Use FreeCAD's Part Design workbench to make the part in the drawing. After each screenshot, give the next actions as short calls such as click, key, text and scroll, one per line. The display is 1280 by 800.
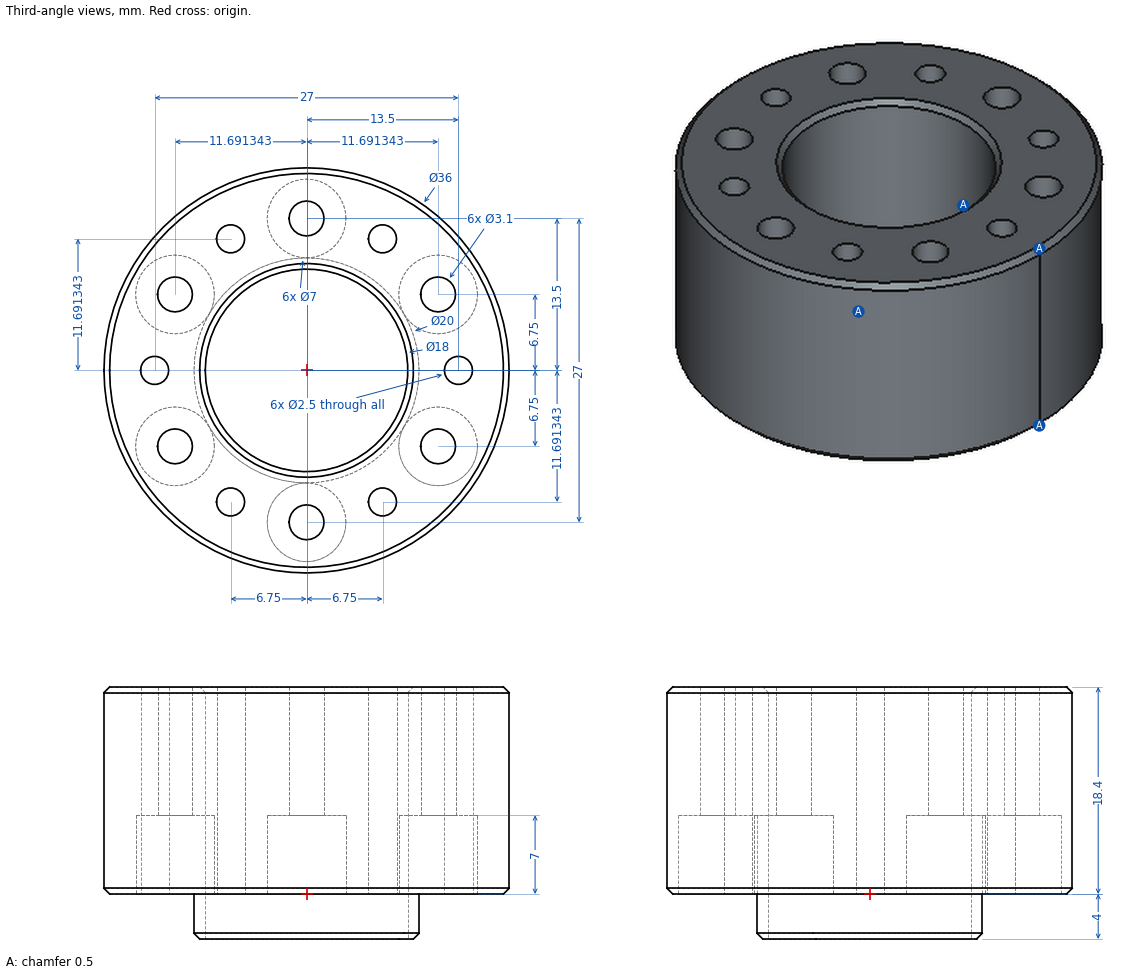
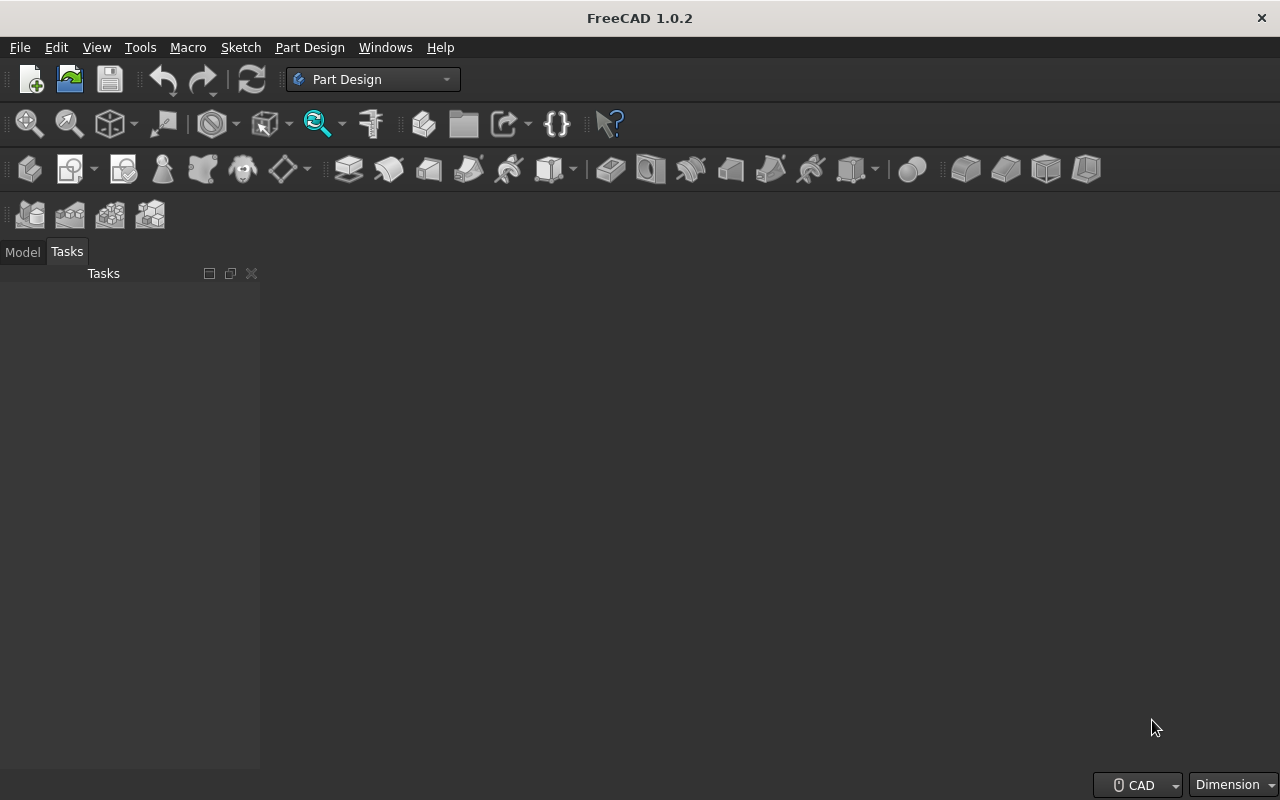
click(30, 80)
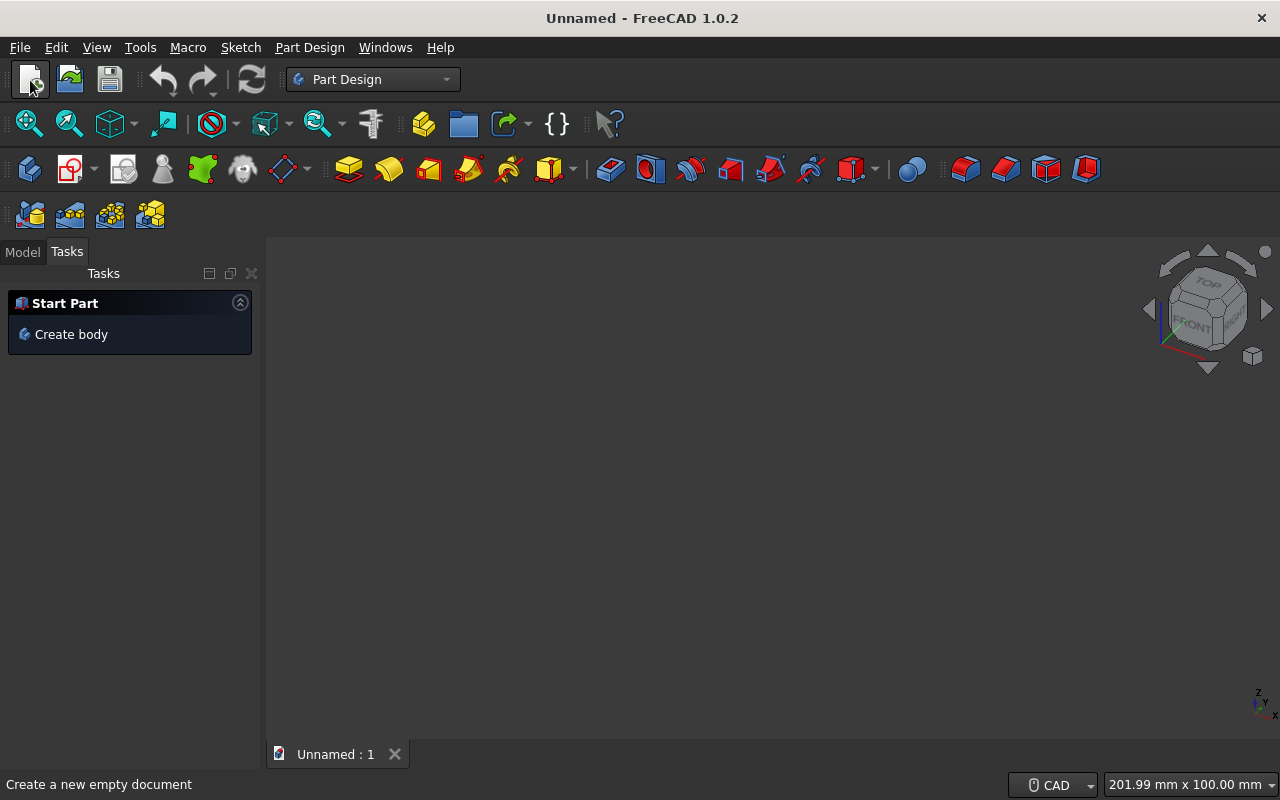
click(70, 170)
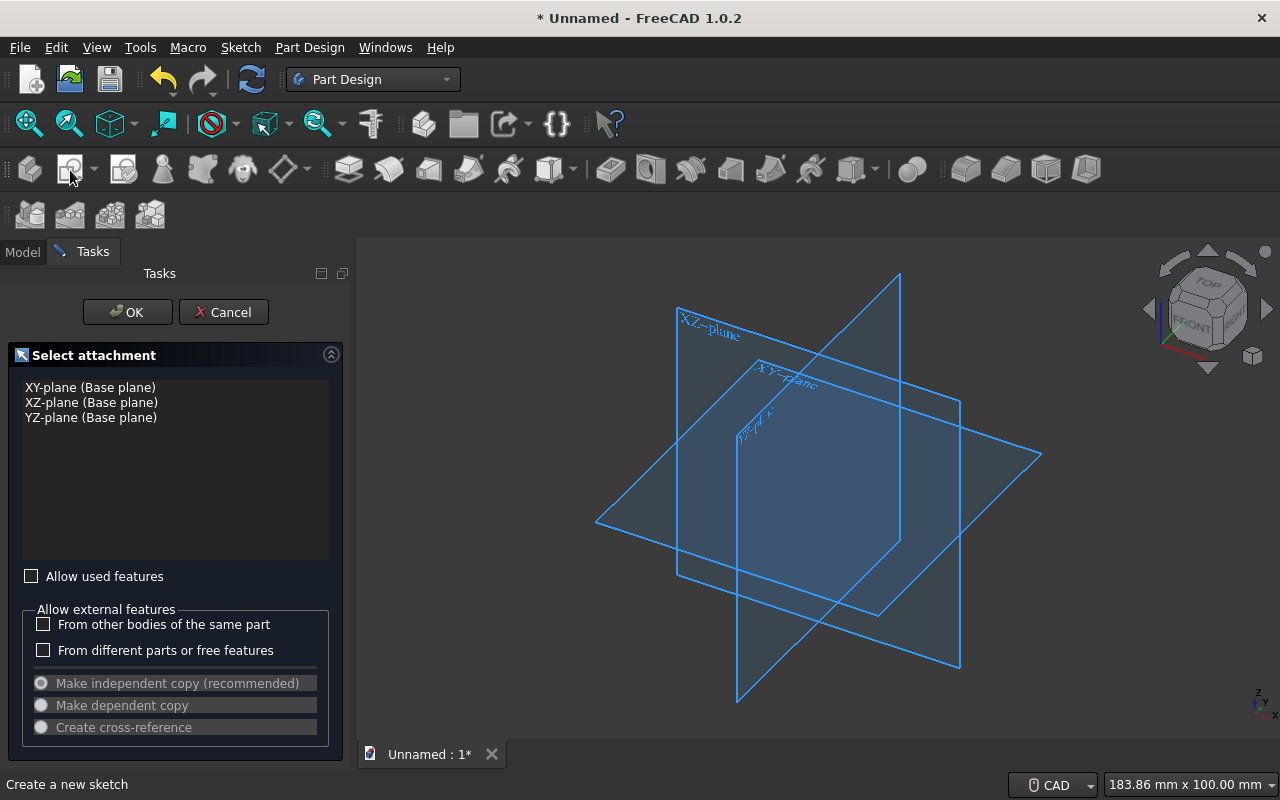
click(82, 388)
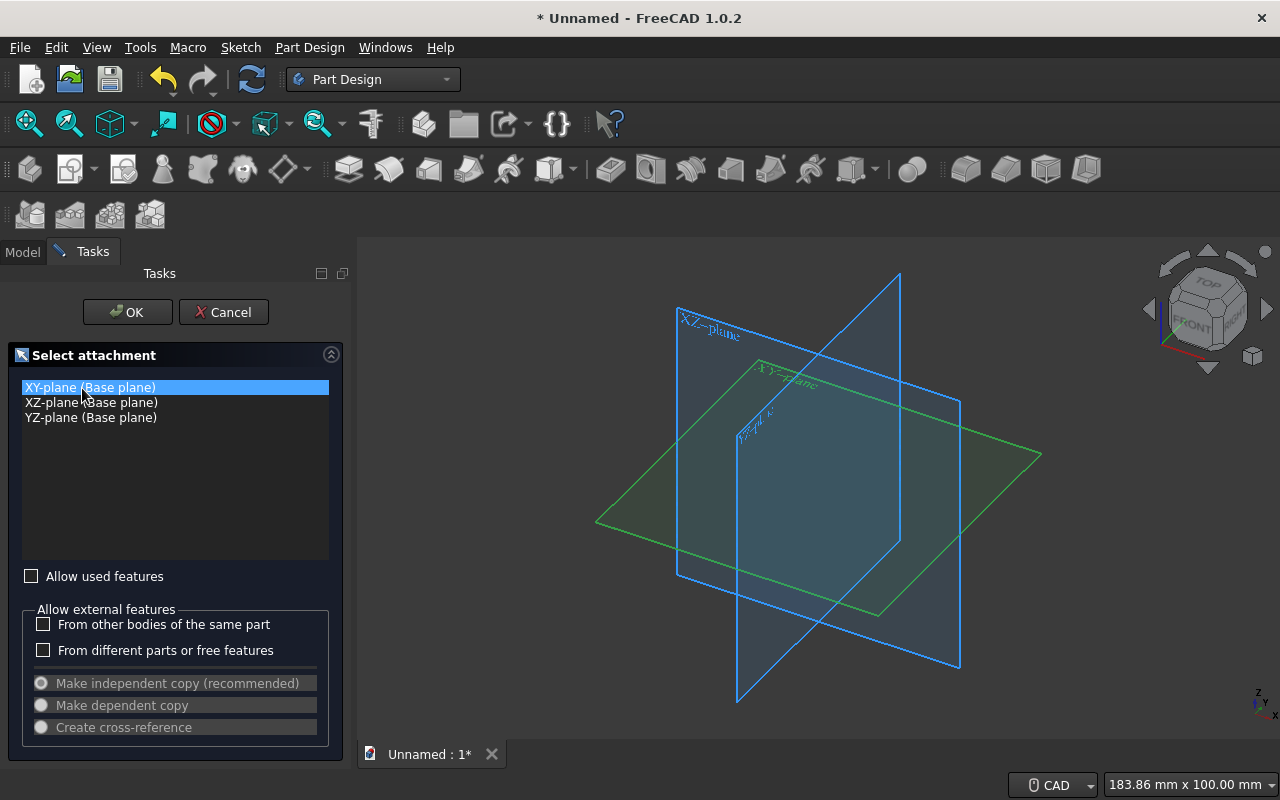
click(128, 312)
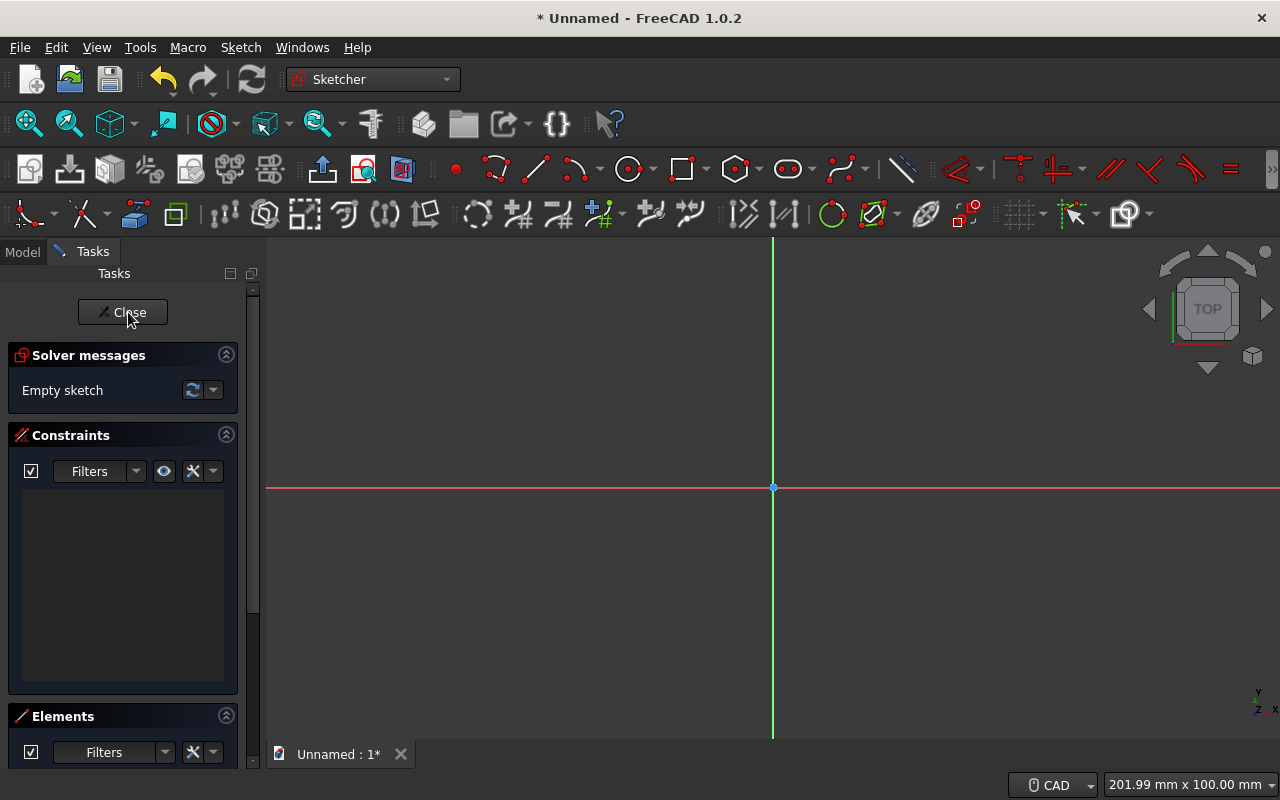
scroll(856, 488, up, 3)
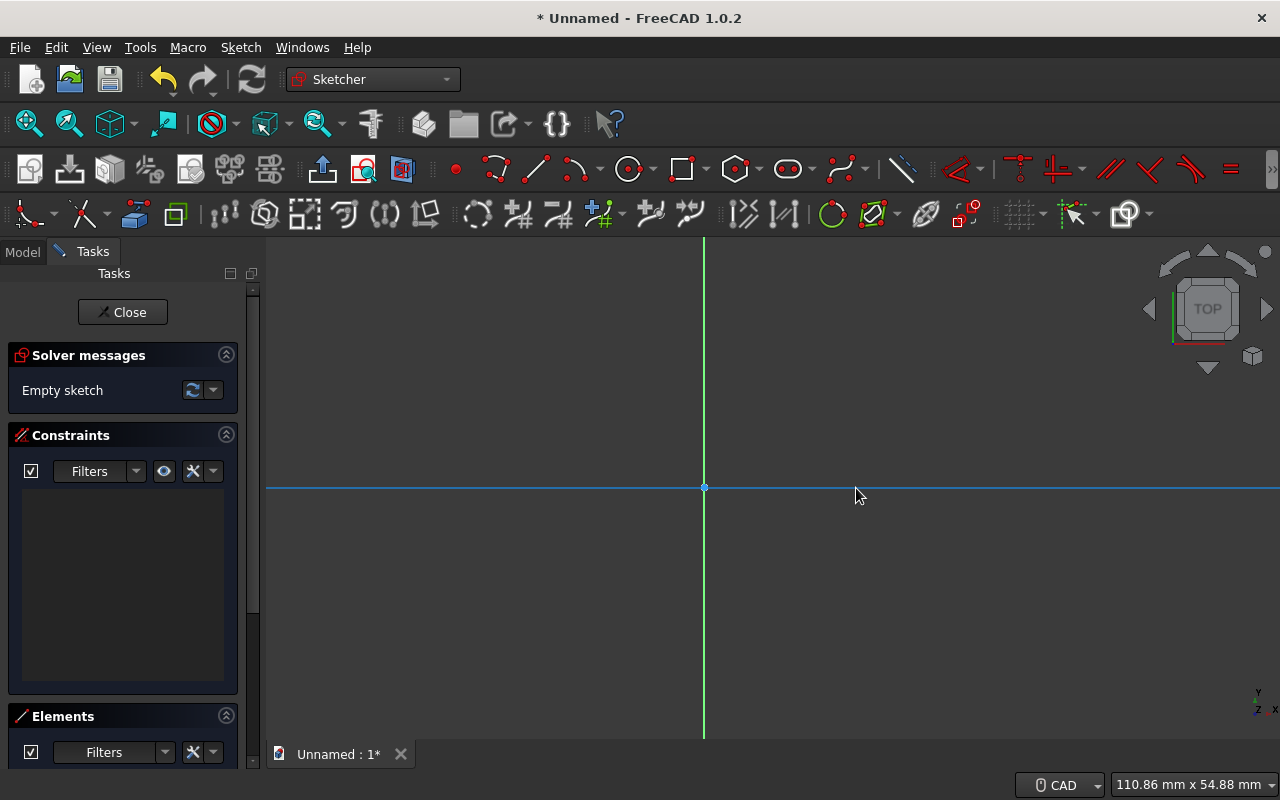
key(g)
key(c)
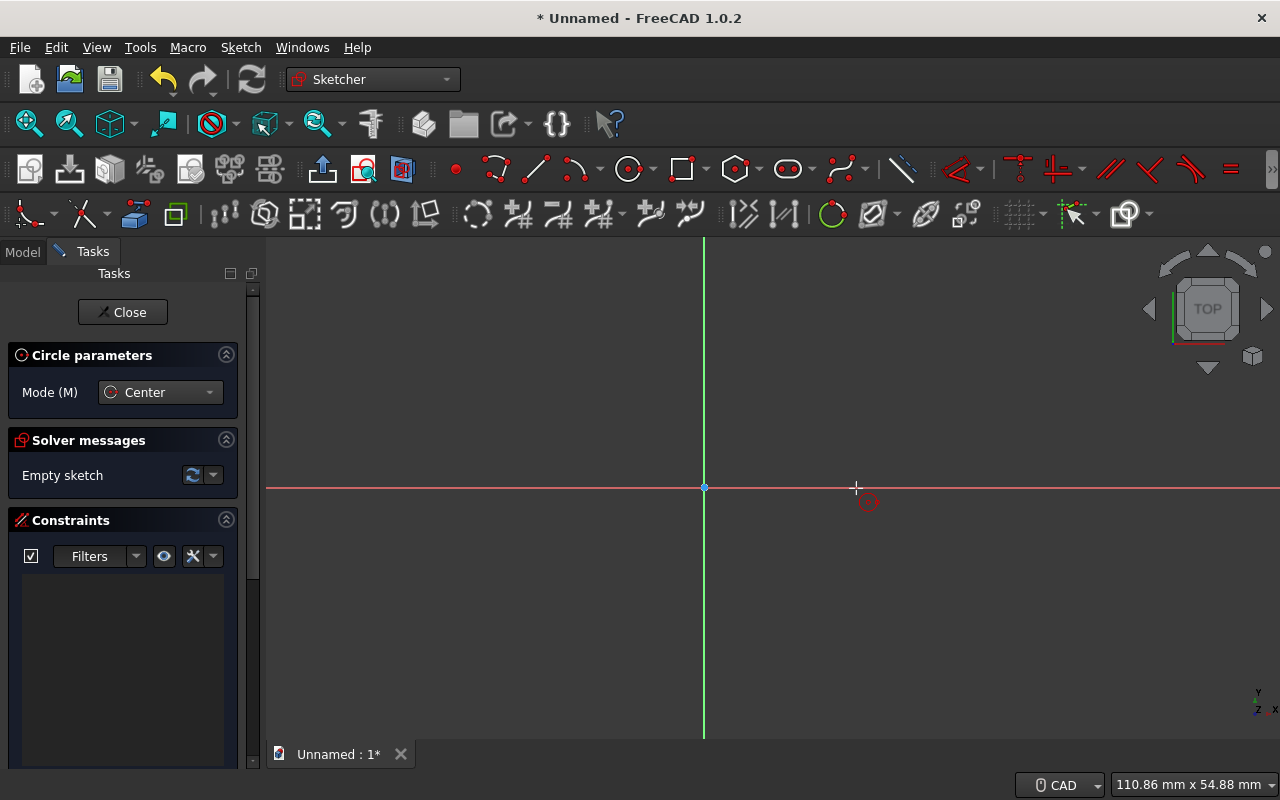
click(704, 488)
click(821, 371)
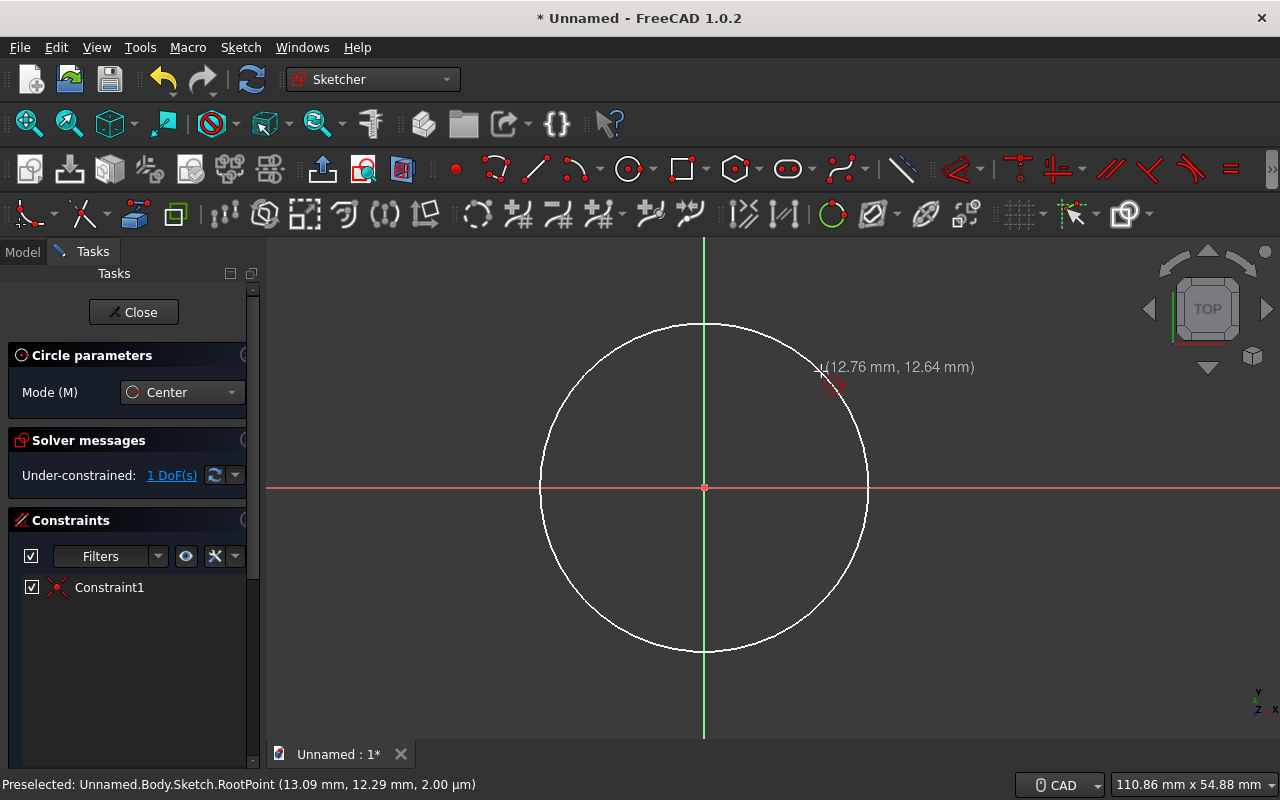
scroll(811, 426, up, 3)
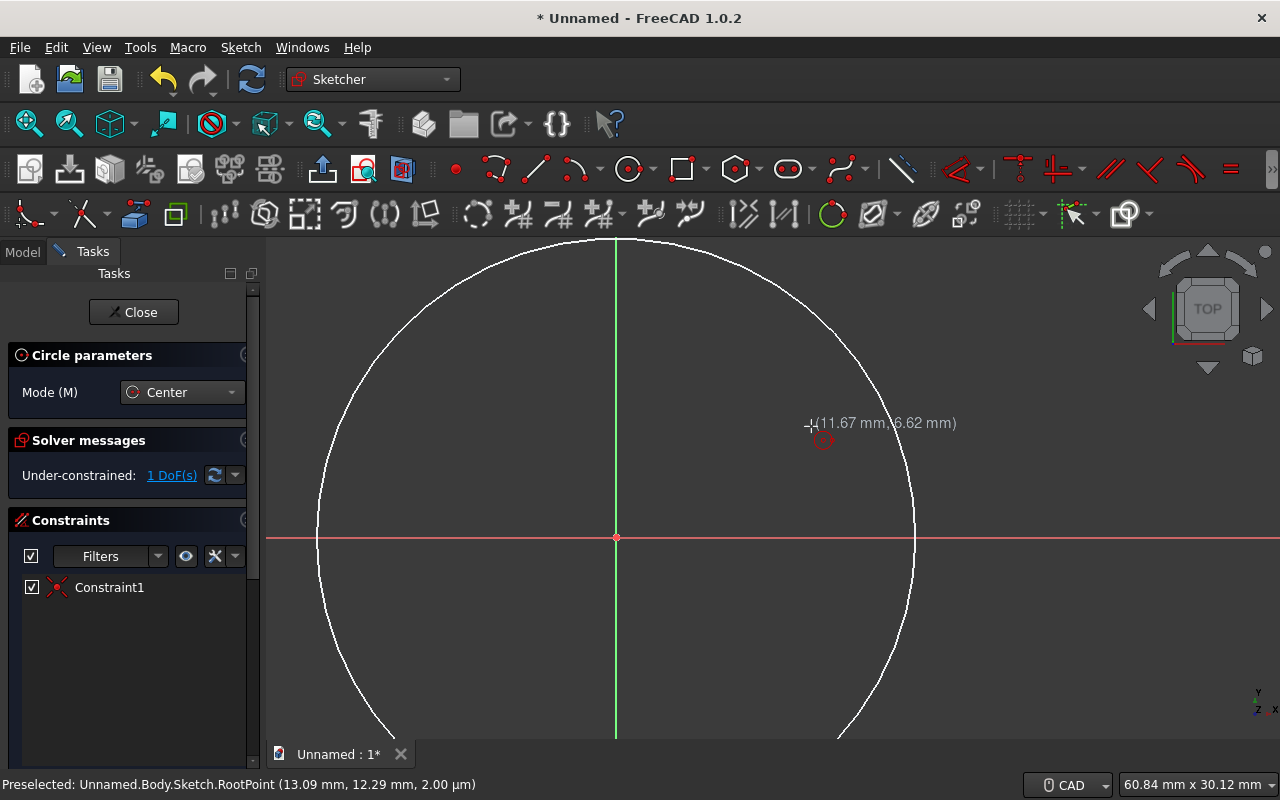
click(811, 425)
click(829, 407)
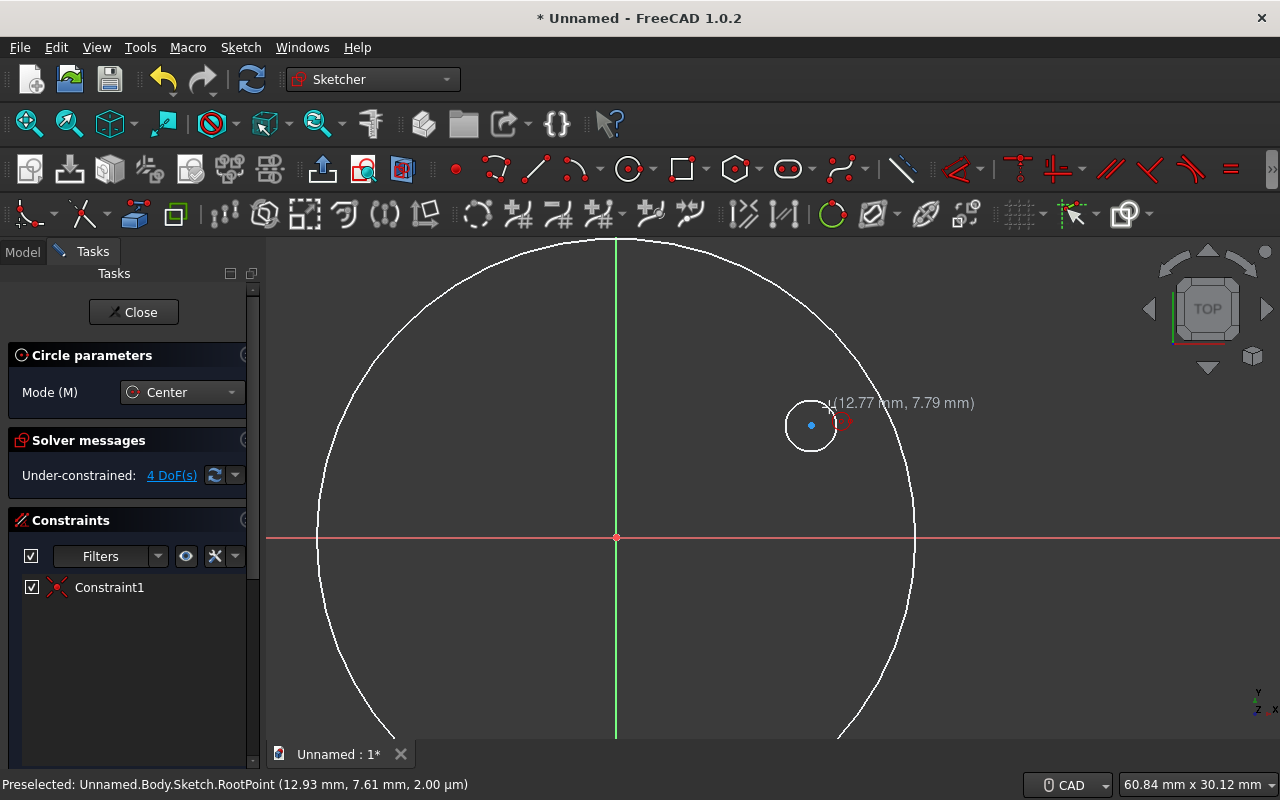
click(616, 313)
click(634, 295)